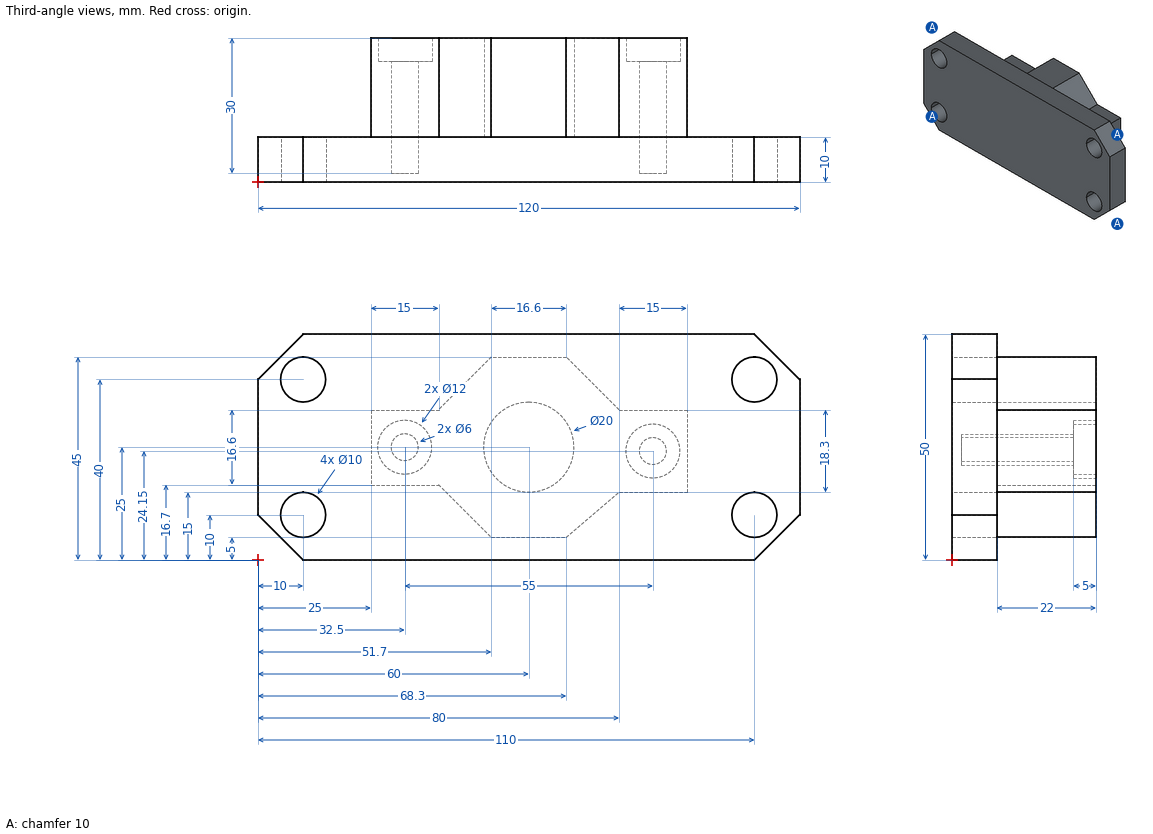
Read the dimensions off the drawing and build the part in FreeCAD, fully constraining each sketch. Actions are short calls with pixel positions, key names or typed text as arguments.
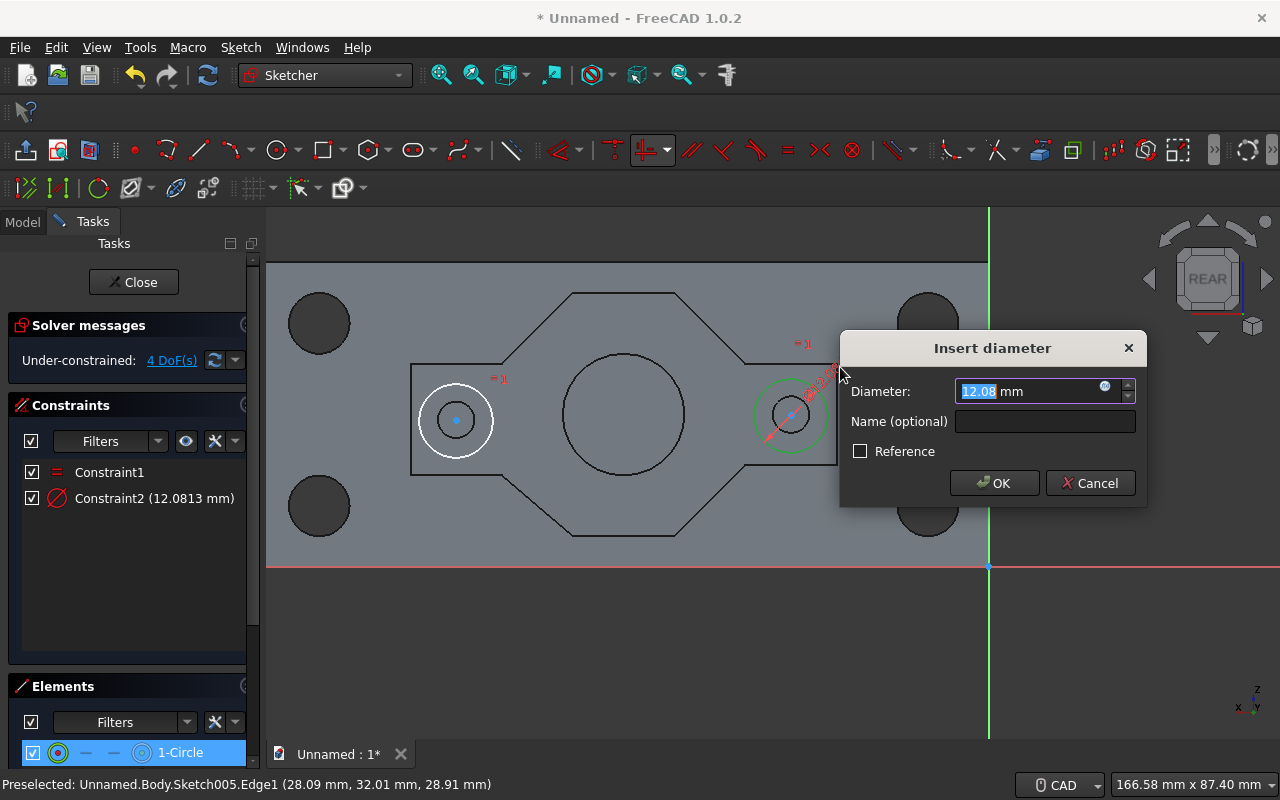
text(12)
key(Return)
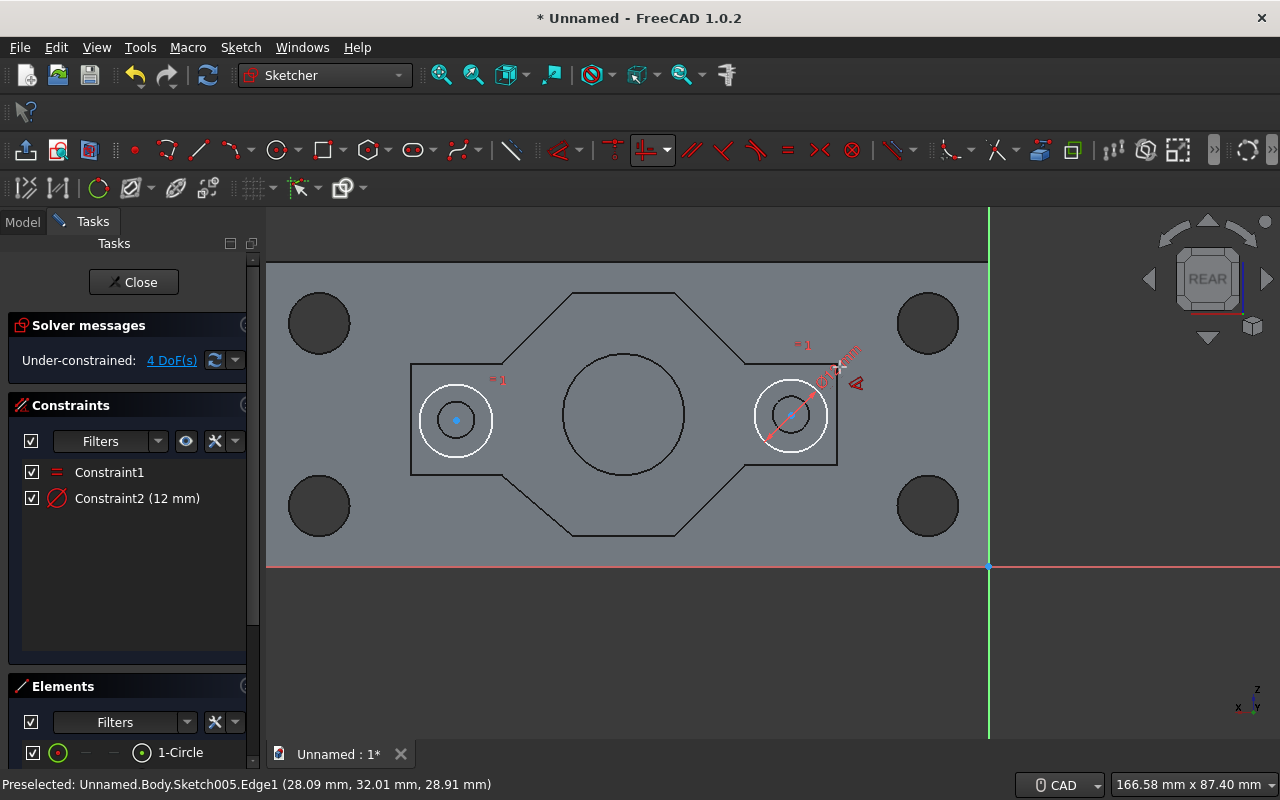
click(791, 416)
click(1023, 491)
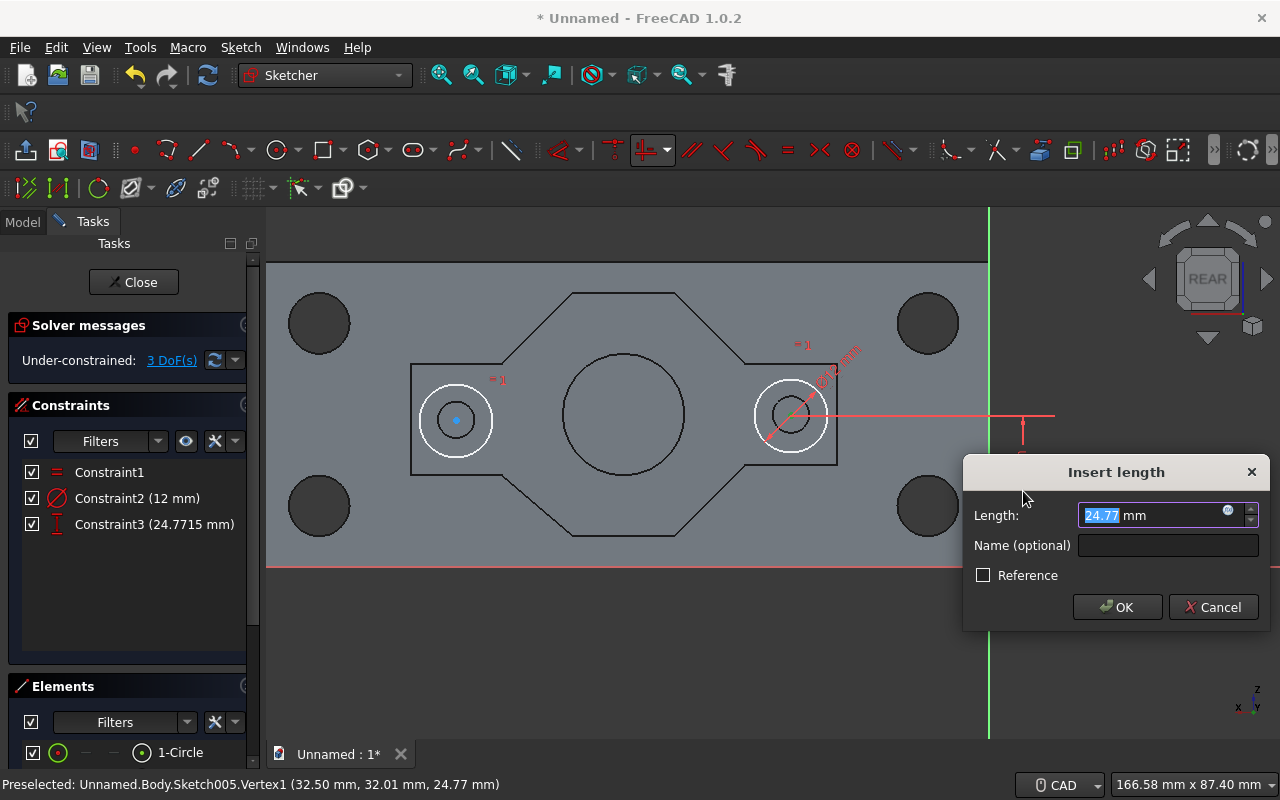
text(25)
key(Return)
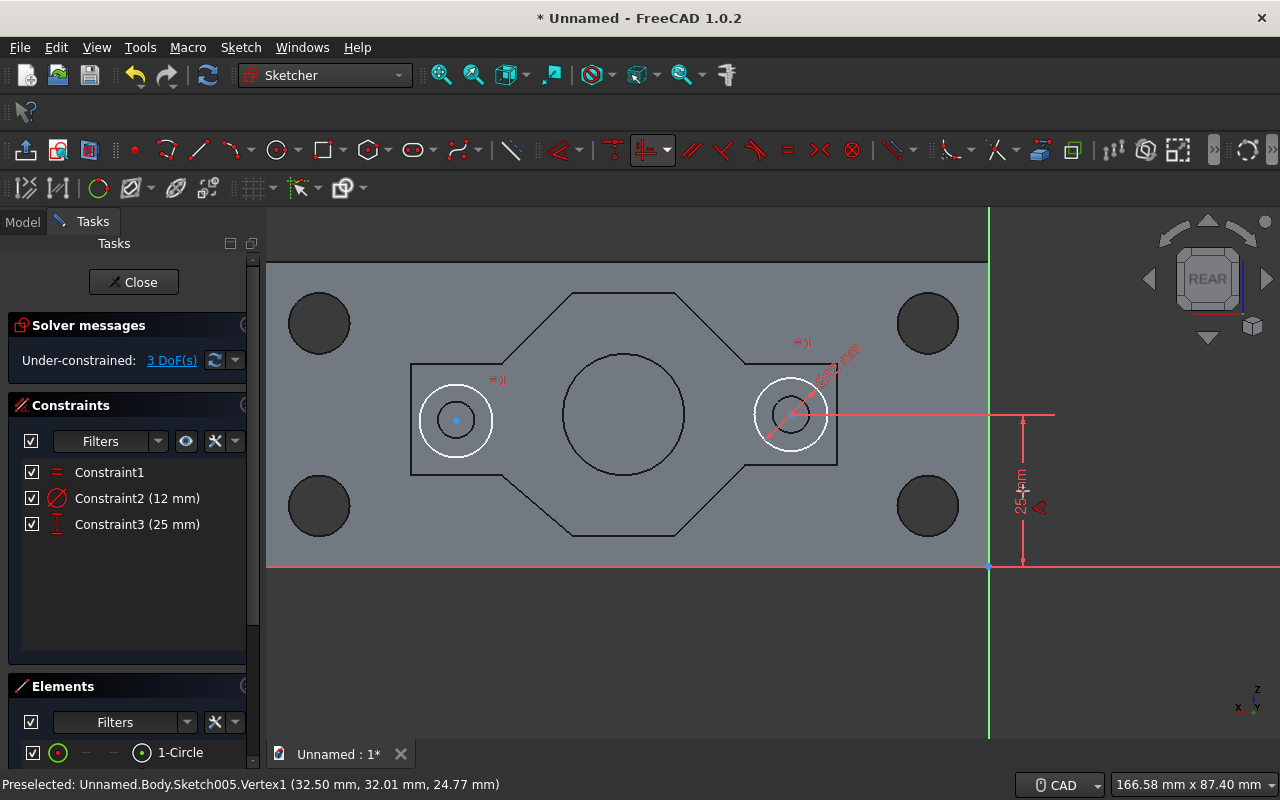
click(791, 415)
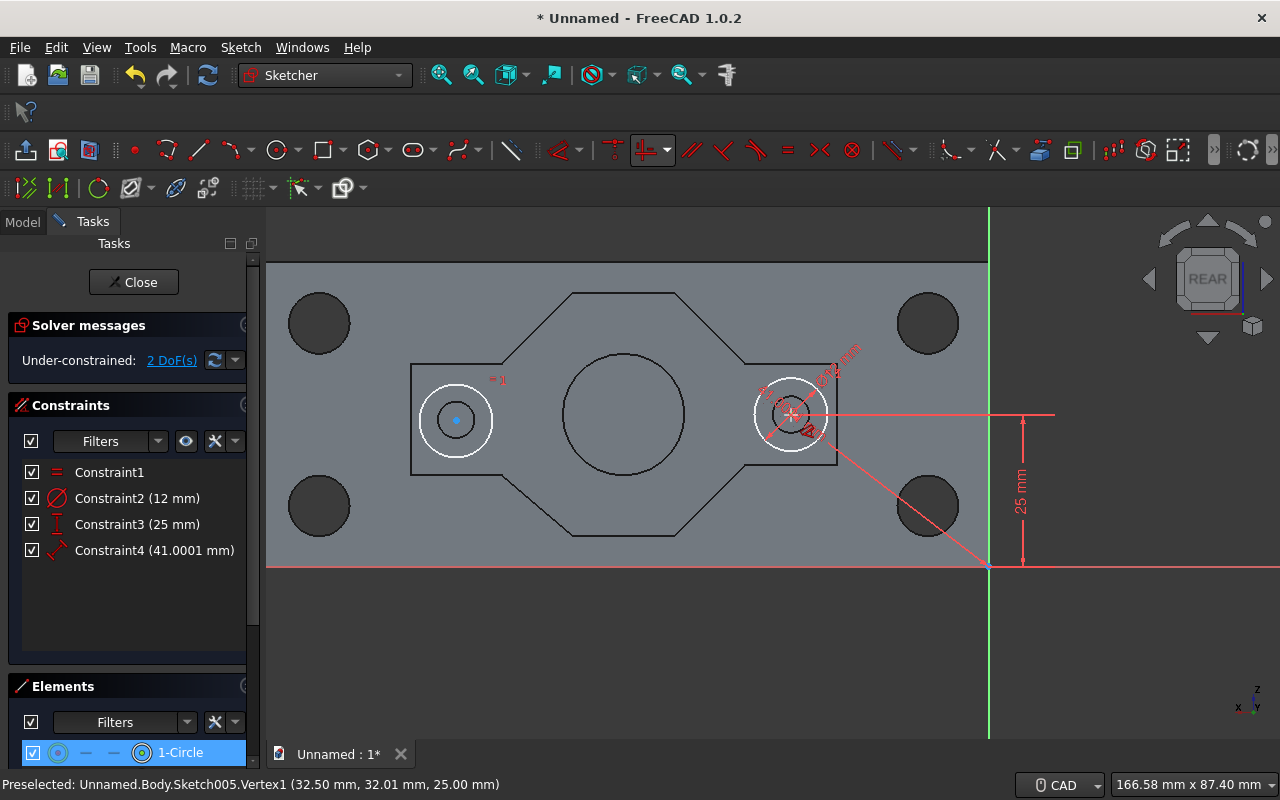
click(456, 421)
click(623, 381)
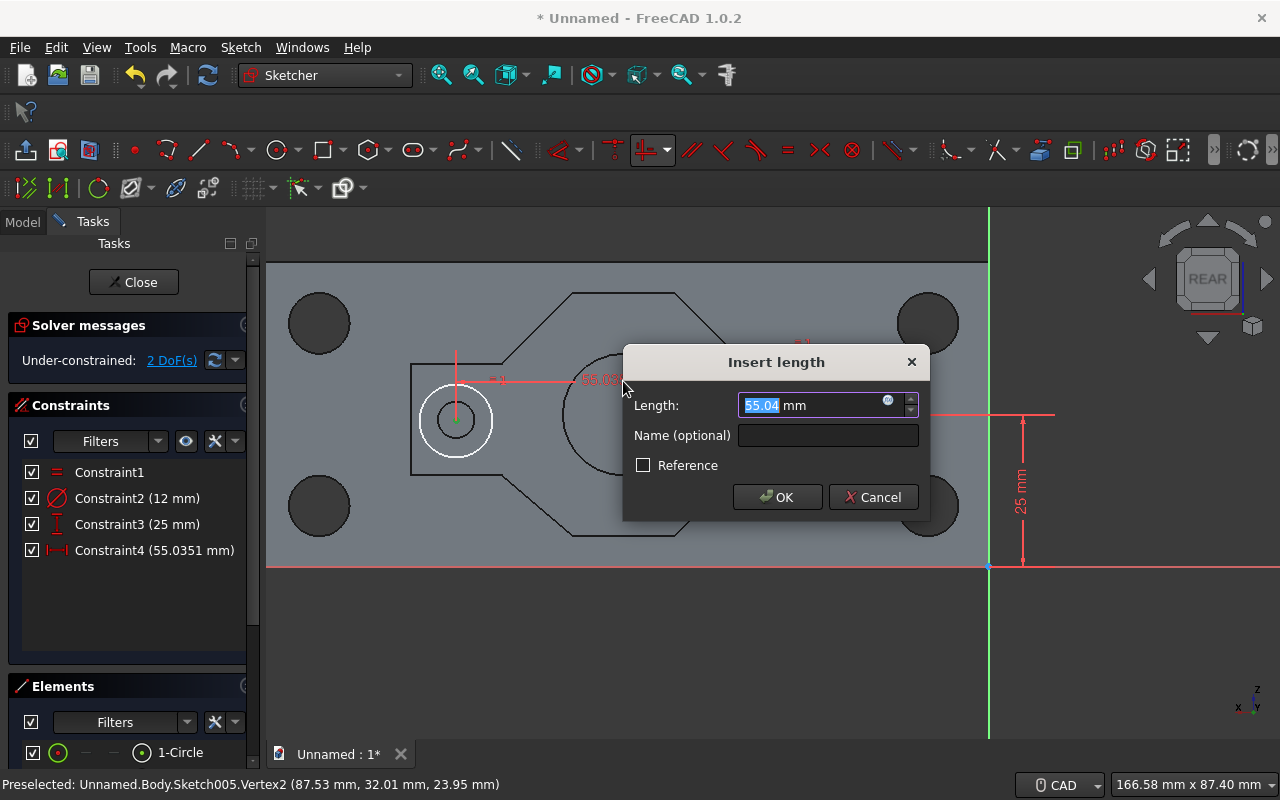
text(55)
key(Return)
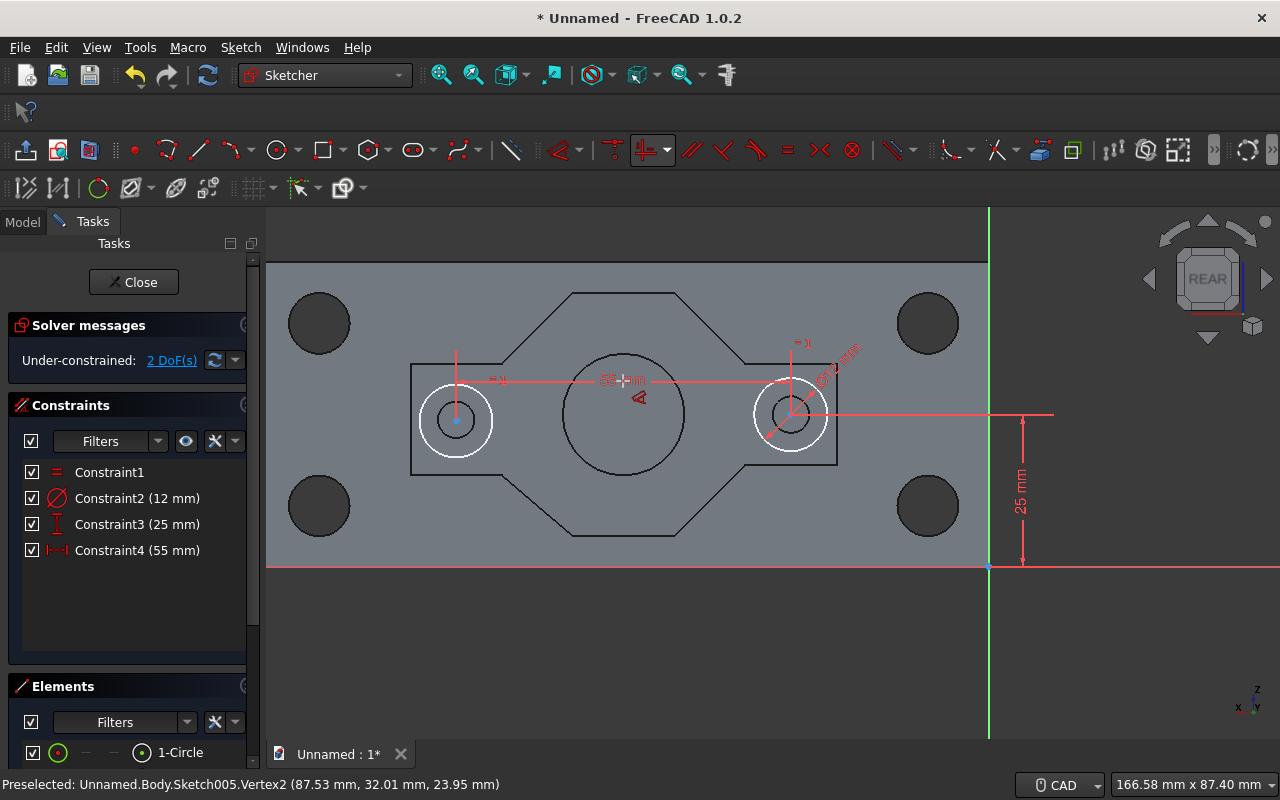
click(791, 415)
click(890, 601)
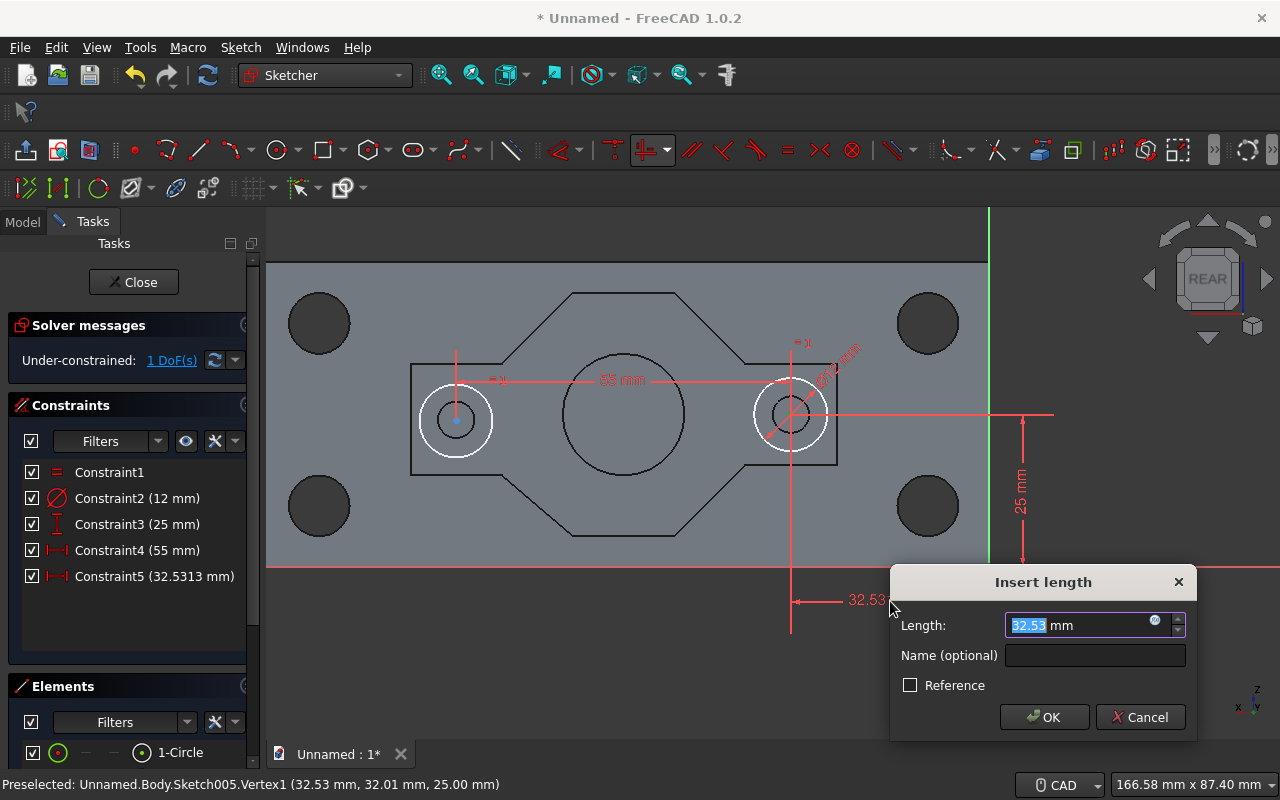
text(32.5)
key(Return)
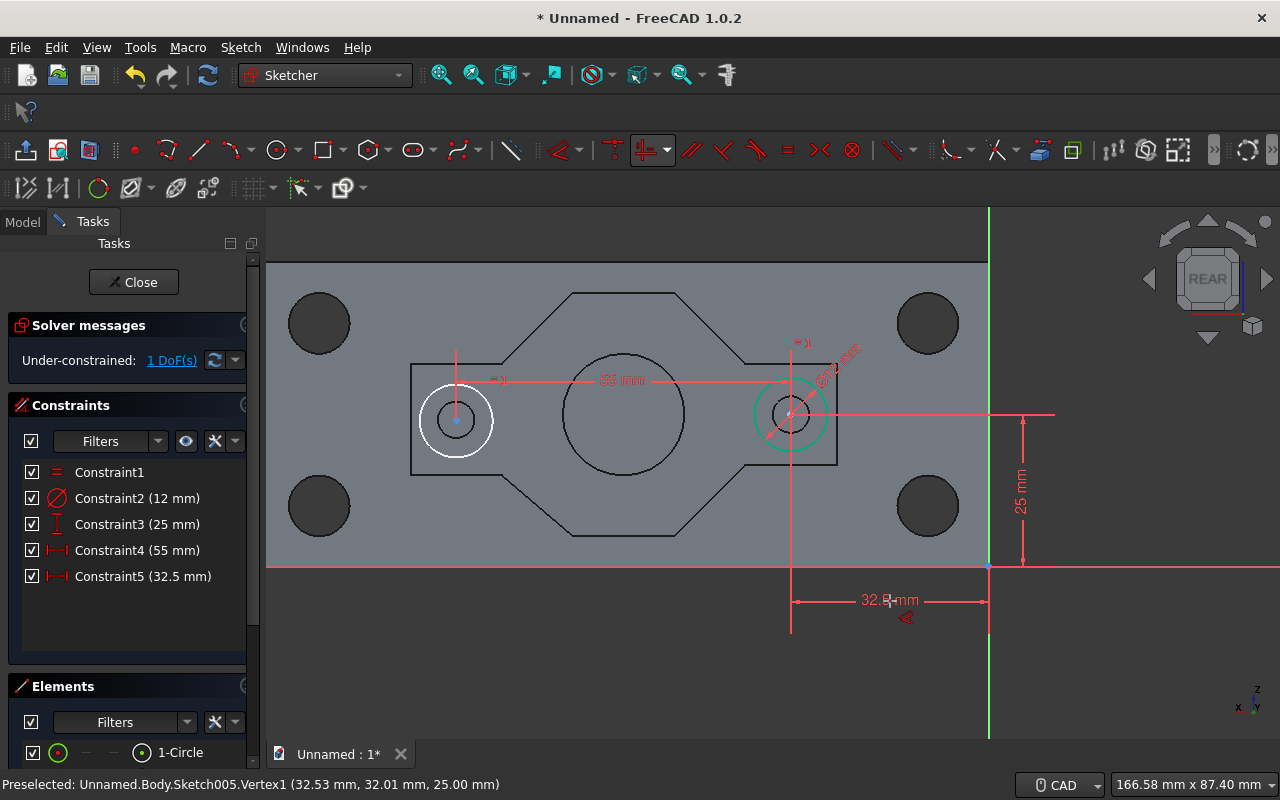
click(456, 421)
click(1023, 460)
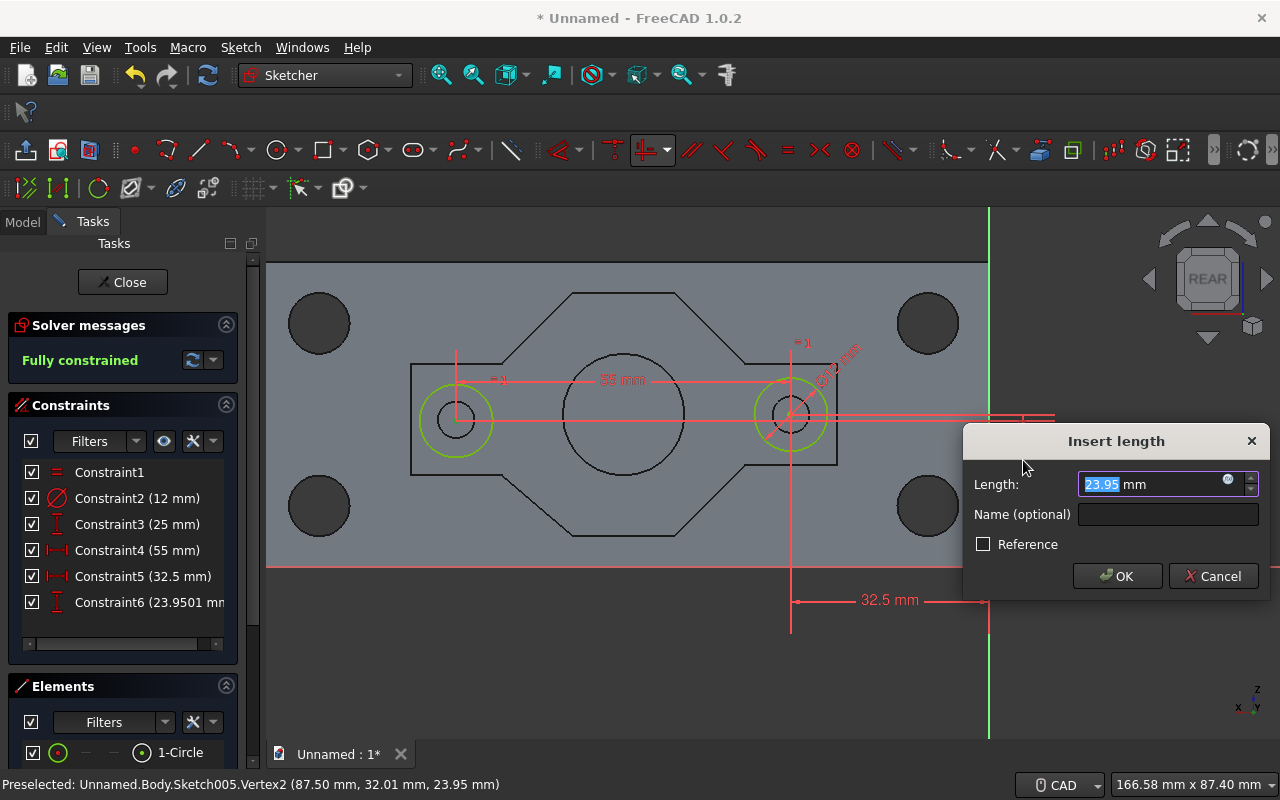
text(24.15)
key(Return)
key(Escape)